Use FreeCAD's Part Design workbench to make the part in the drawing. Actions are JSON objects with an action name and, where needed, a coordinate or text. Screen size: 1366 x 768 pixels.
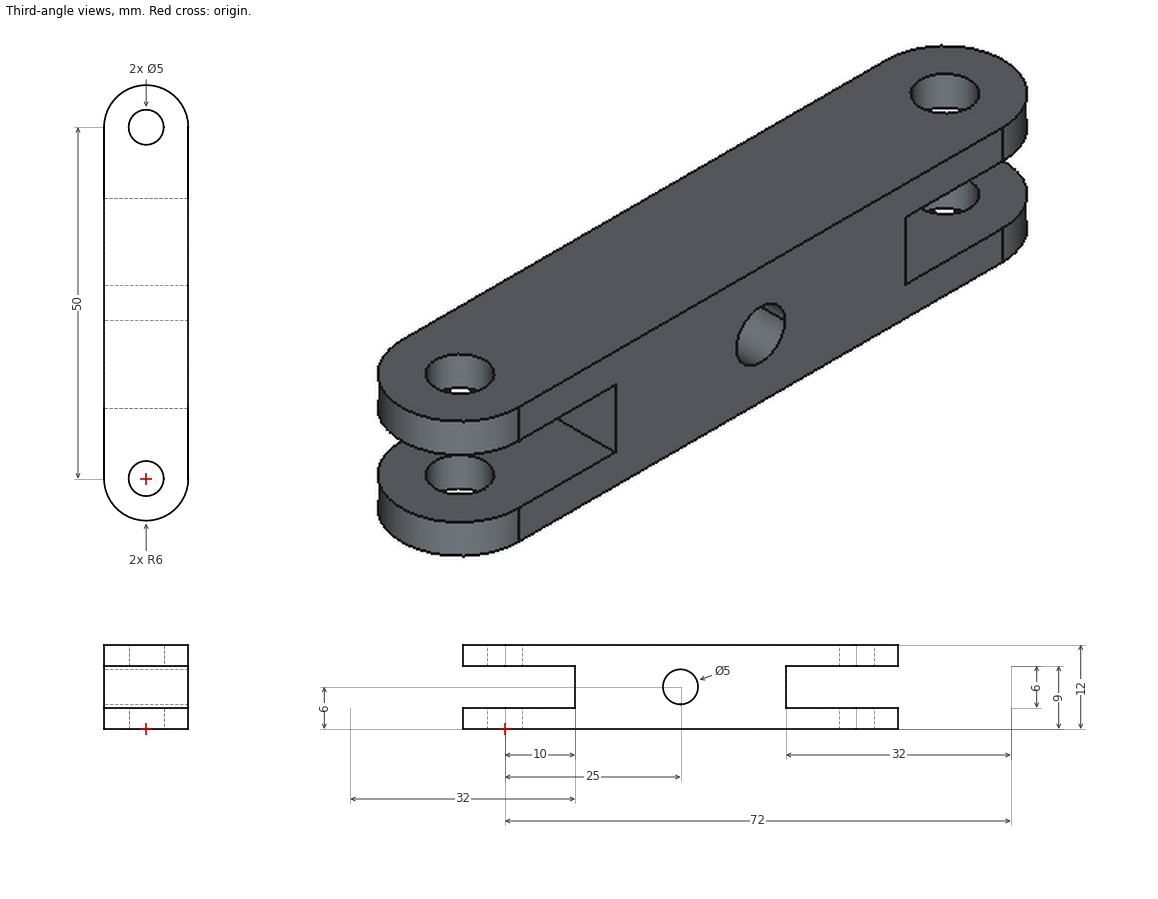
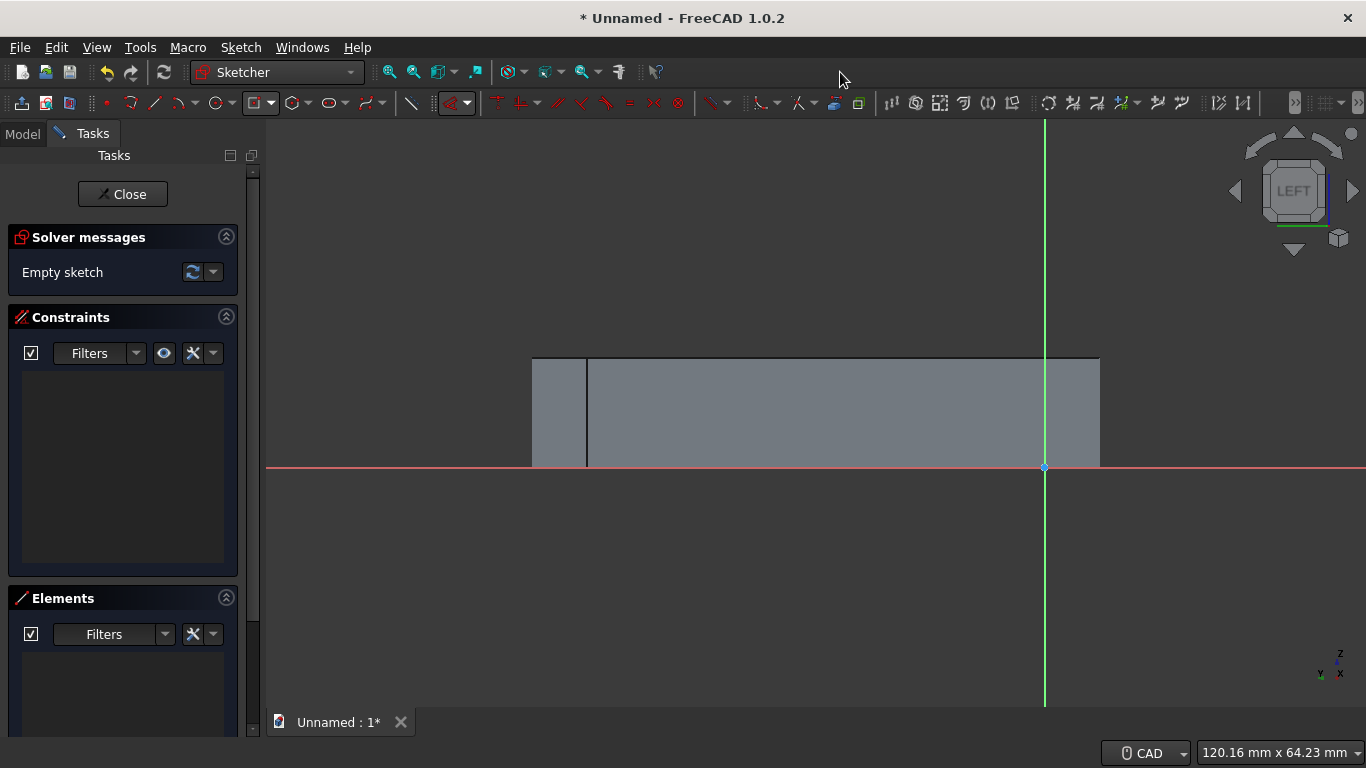
{"action": "scroll", "coordinate": [438, 351], "scroll_direction": "down", "scroll_amount": 1}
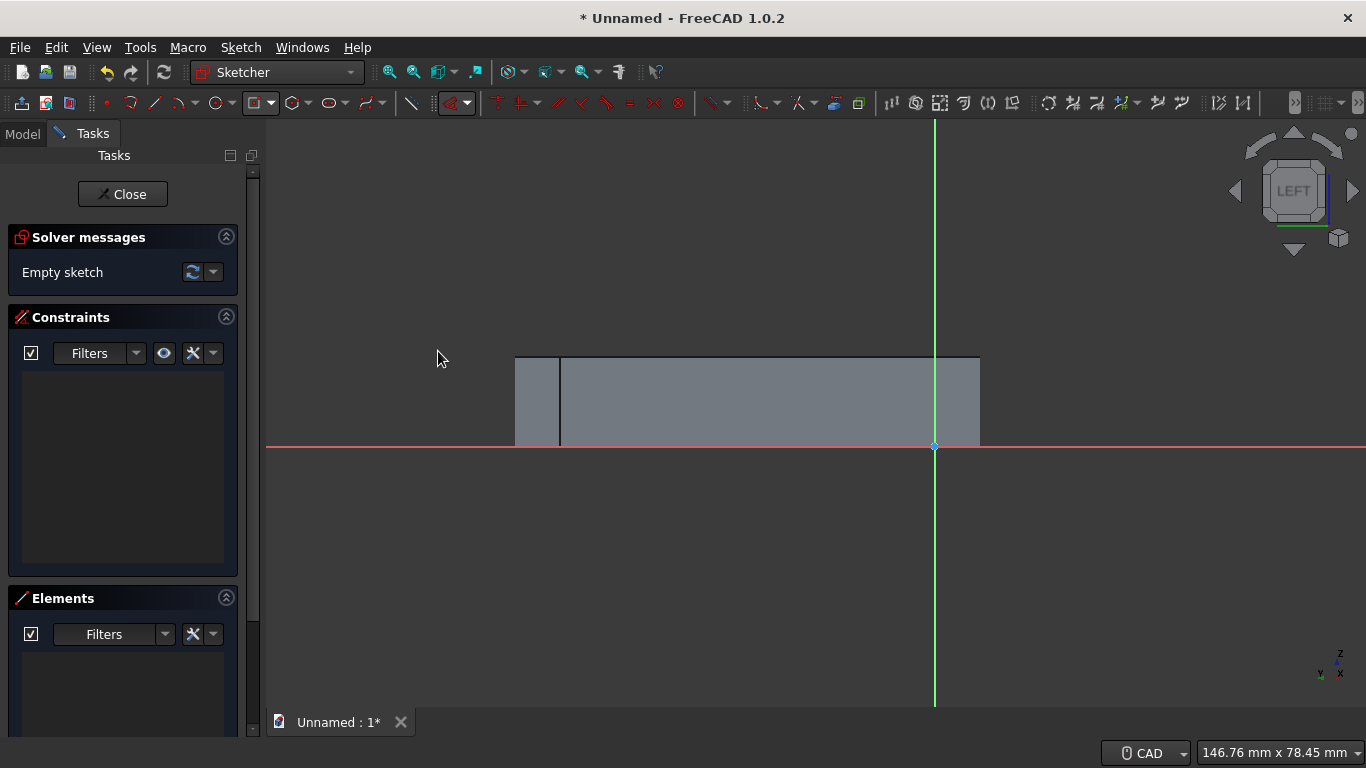
{"action": "key", "text": "g r"}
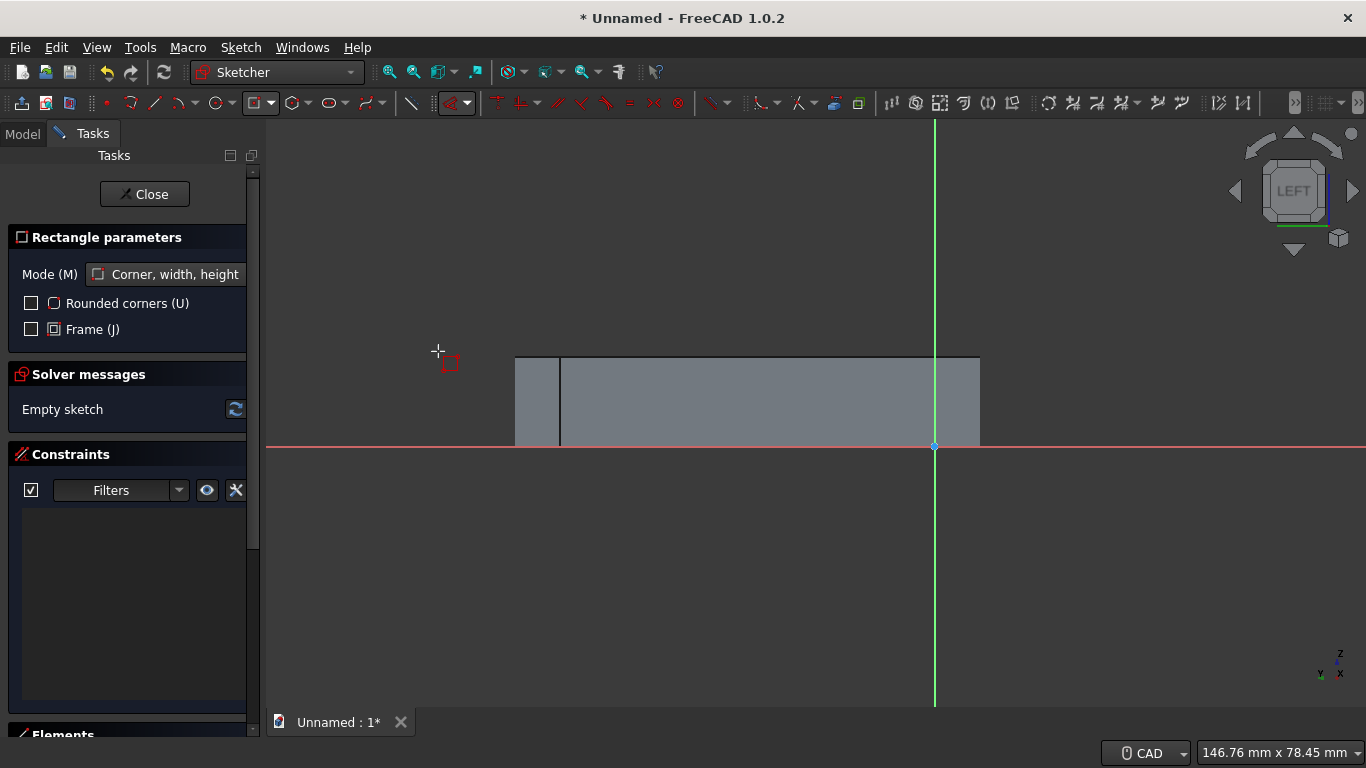
{"action": "left_click", "coordinate": [395, 379]}
{"action": "left_click", "coordinate": [635, 424]}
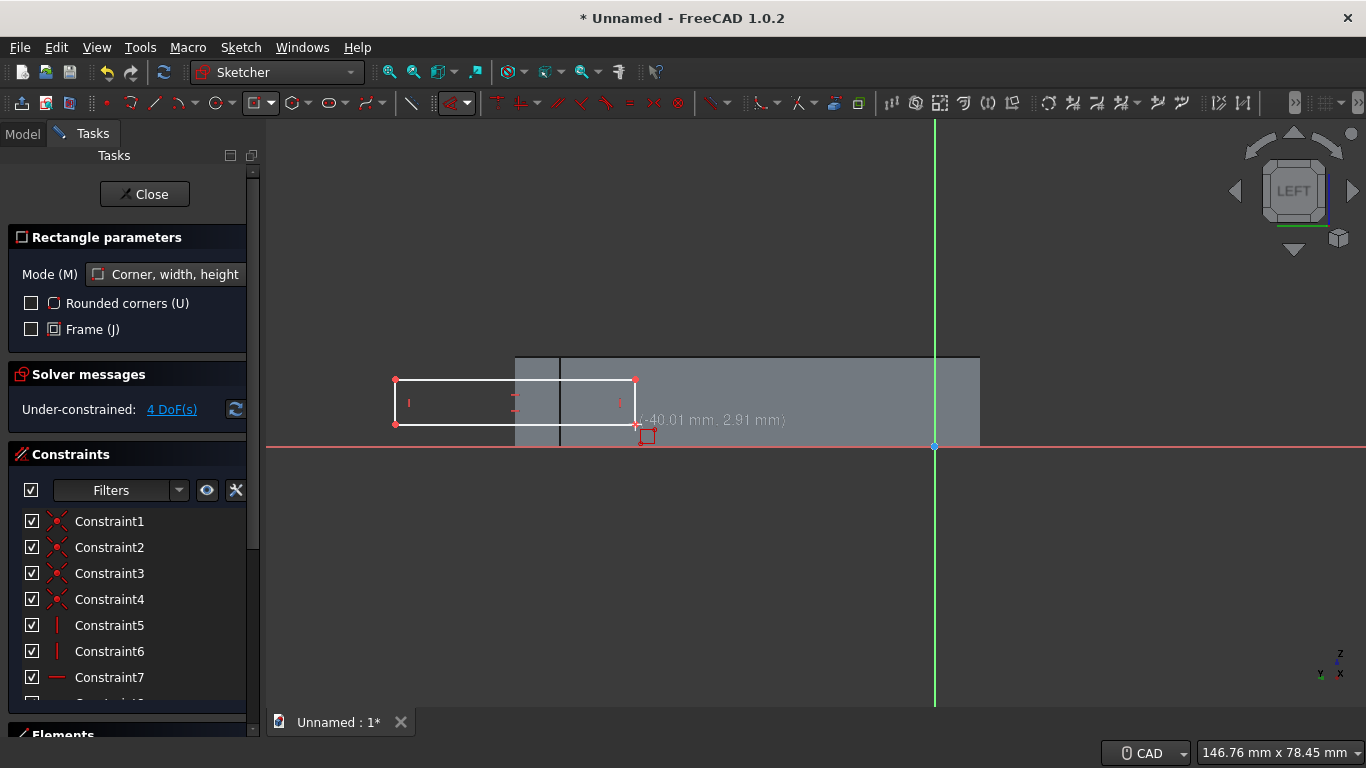
{"action": "left_click", "coordinate": [860, 379]}
{"action": "left_click", "coordinate": [1100, 424]}
{"action": "key", "text": "Escape"}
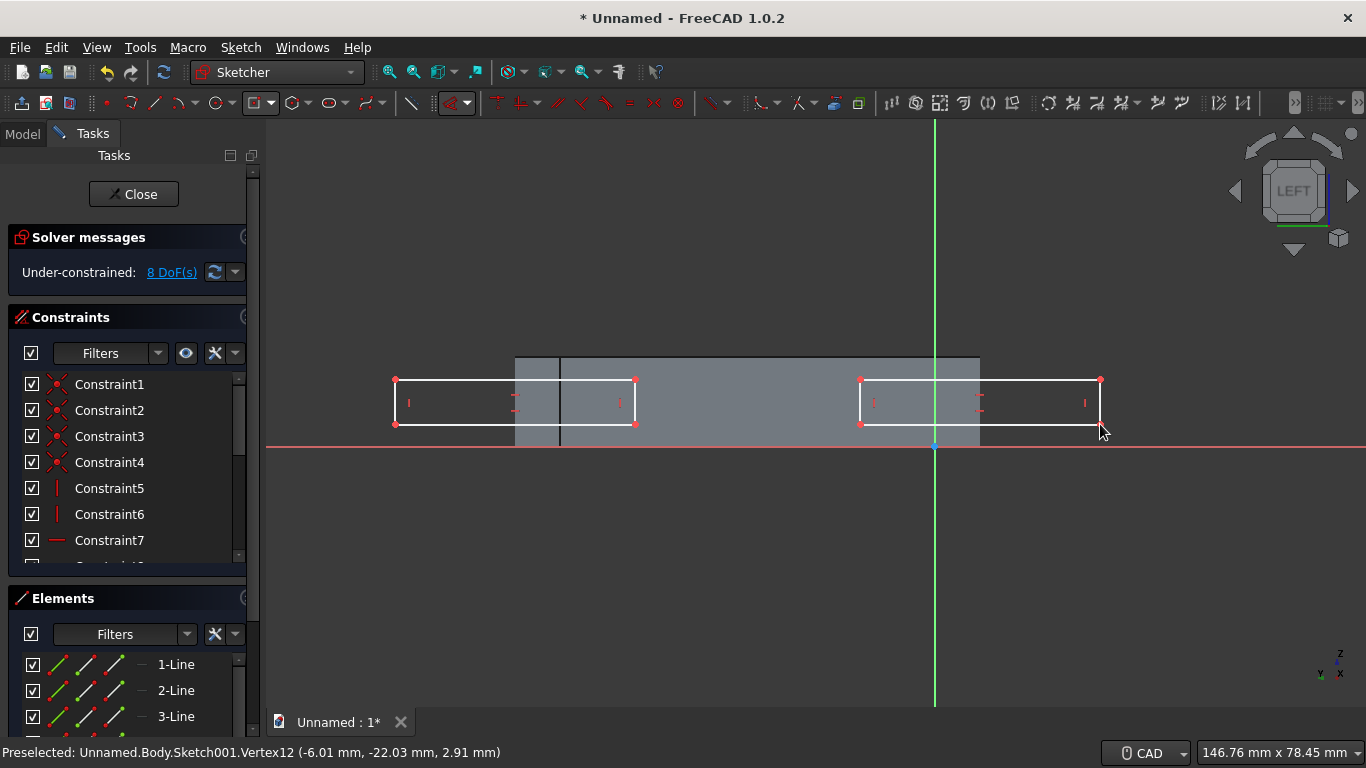
{"action": "left_click", "coordinate": [395, 394]}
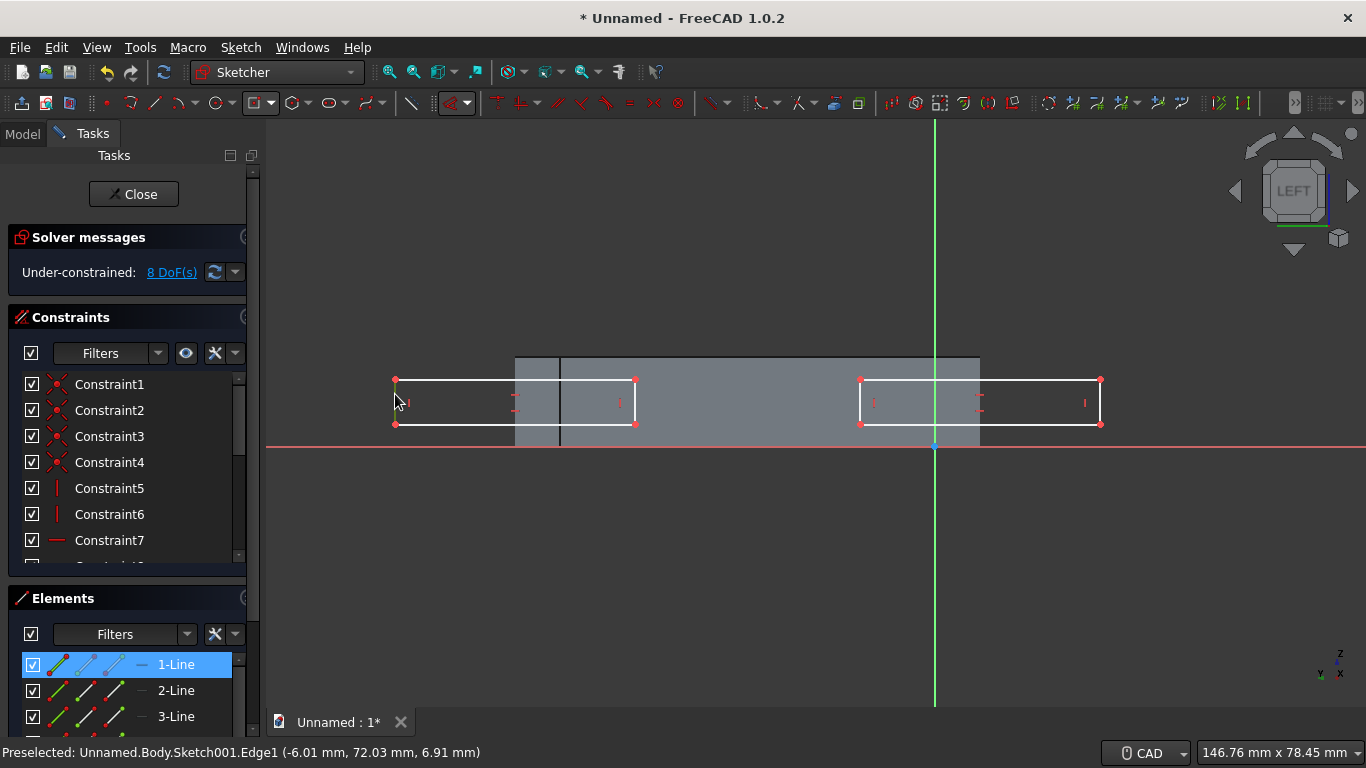
{"action": "key", "text": "i"}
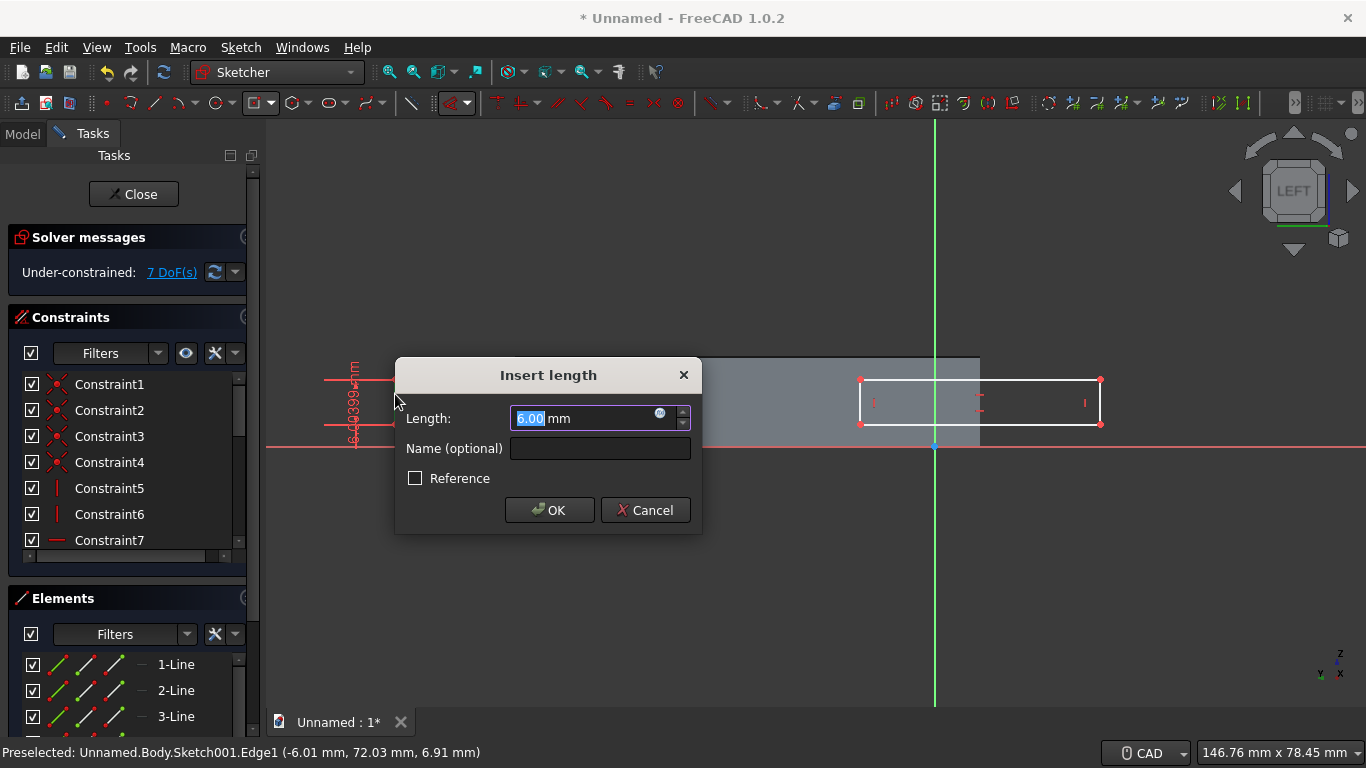
{"action": "type", "text": "6"}
{"action": "key", "text": "Return"}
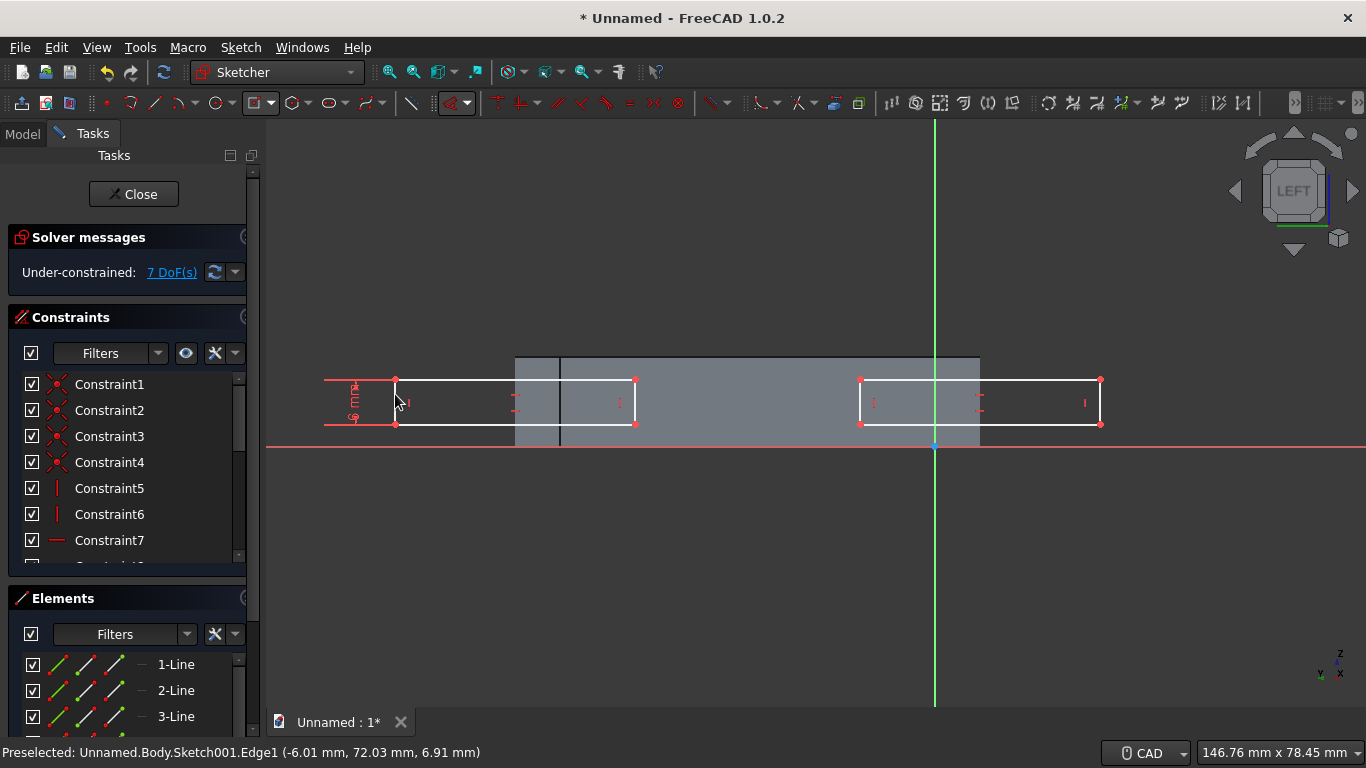
{"action": "left_click", "coordinate": [860, 394]}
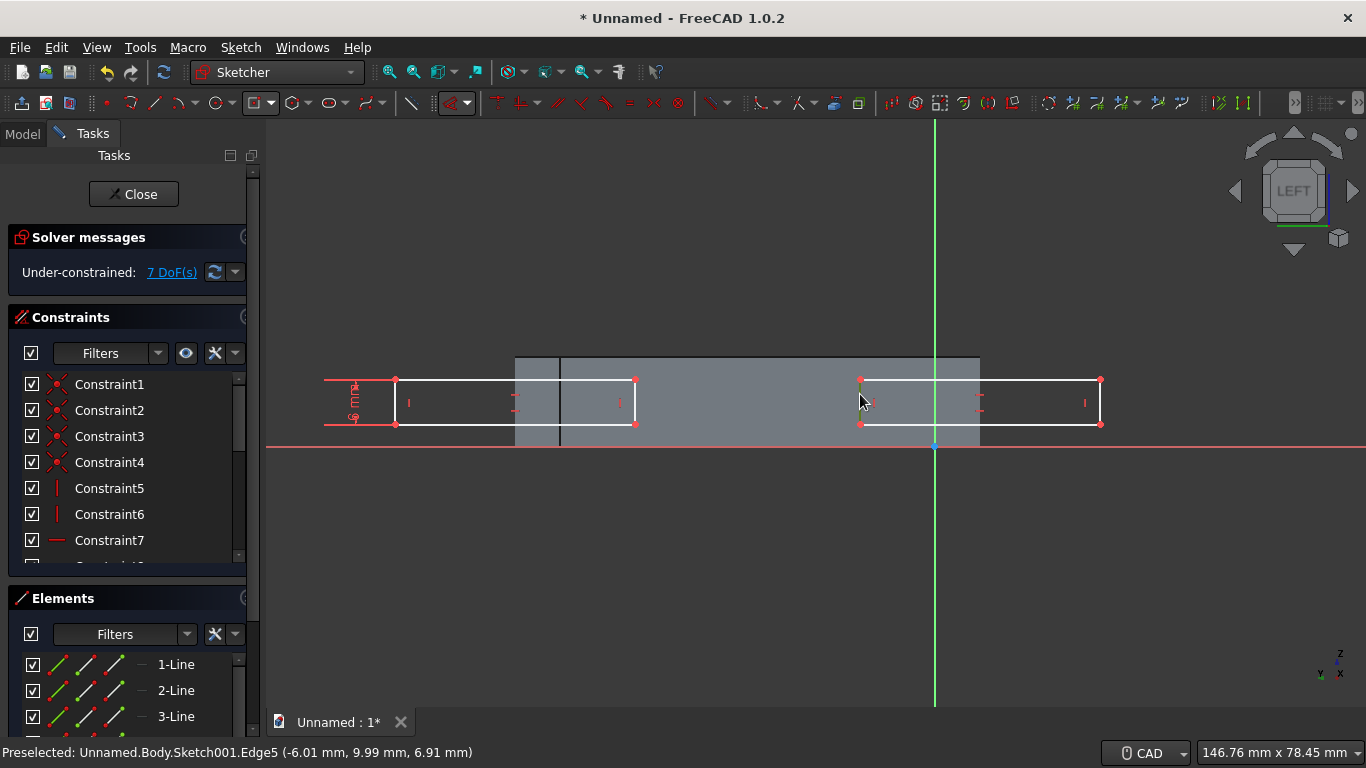
{"action": "key", "text": "i"}